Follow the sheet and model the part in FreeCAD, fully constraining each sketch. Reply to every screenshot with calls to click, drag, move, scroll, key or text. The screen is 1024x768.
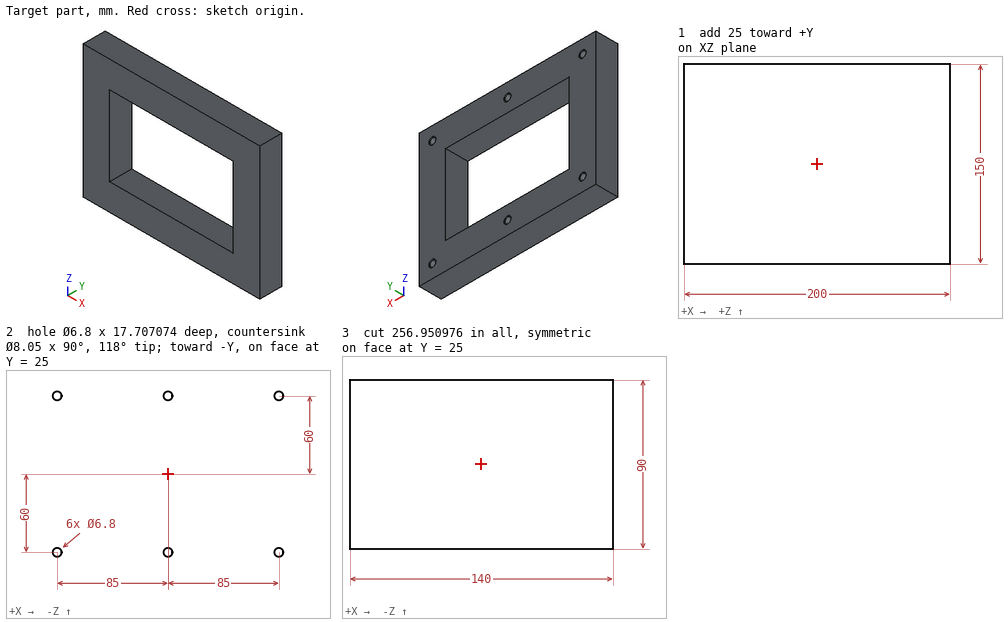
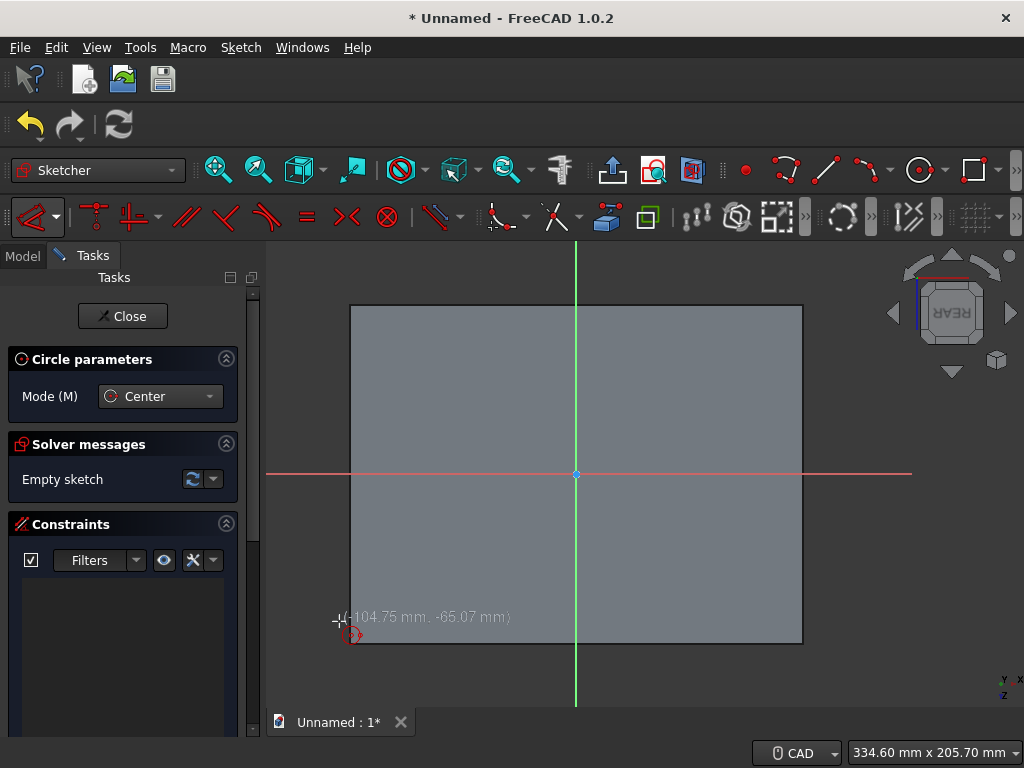
click(384, 610)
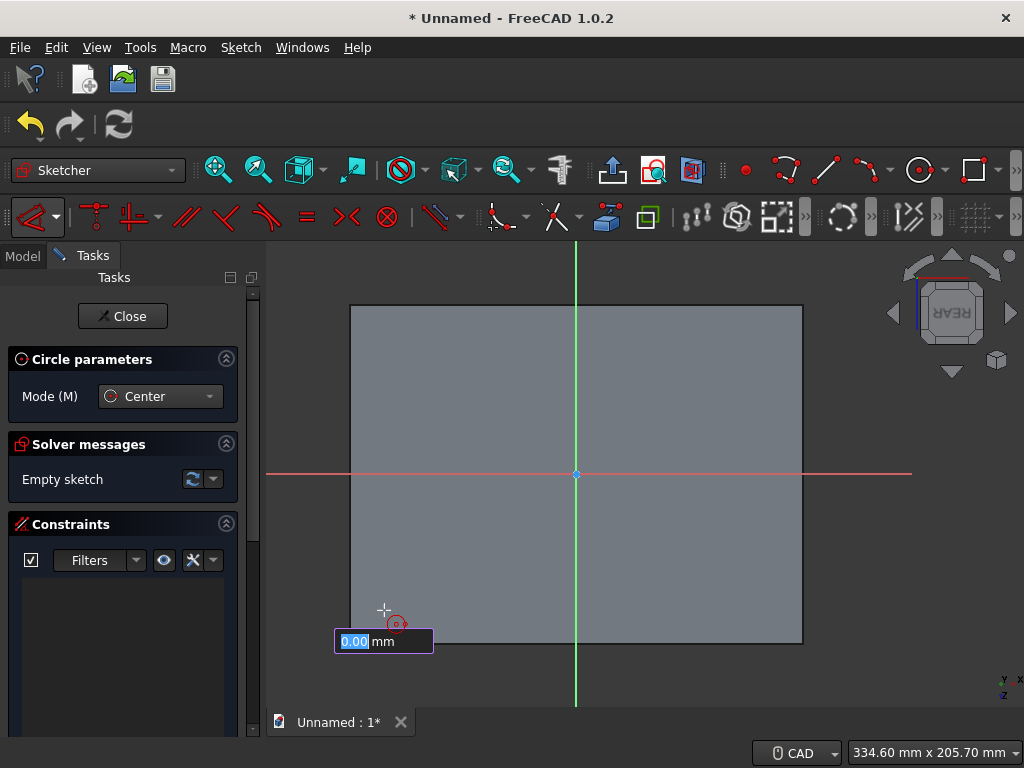
scroll(389, 605, up, 4)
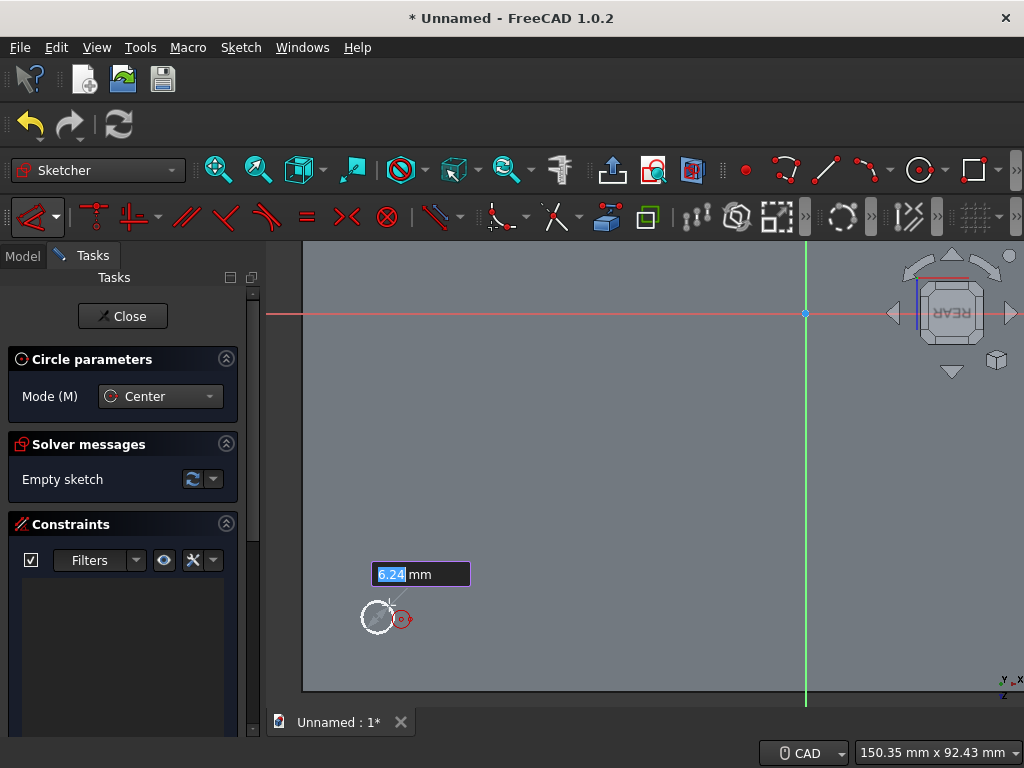
click(389, 604)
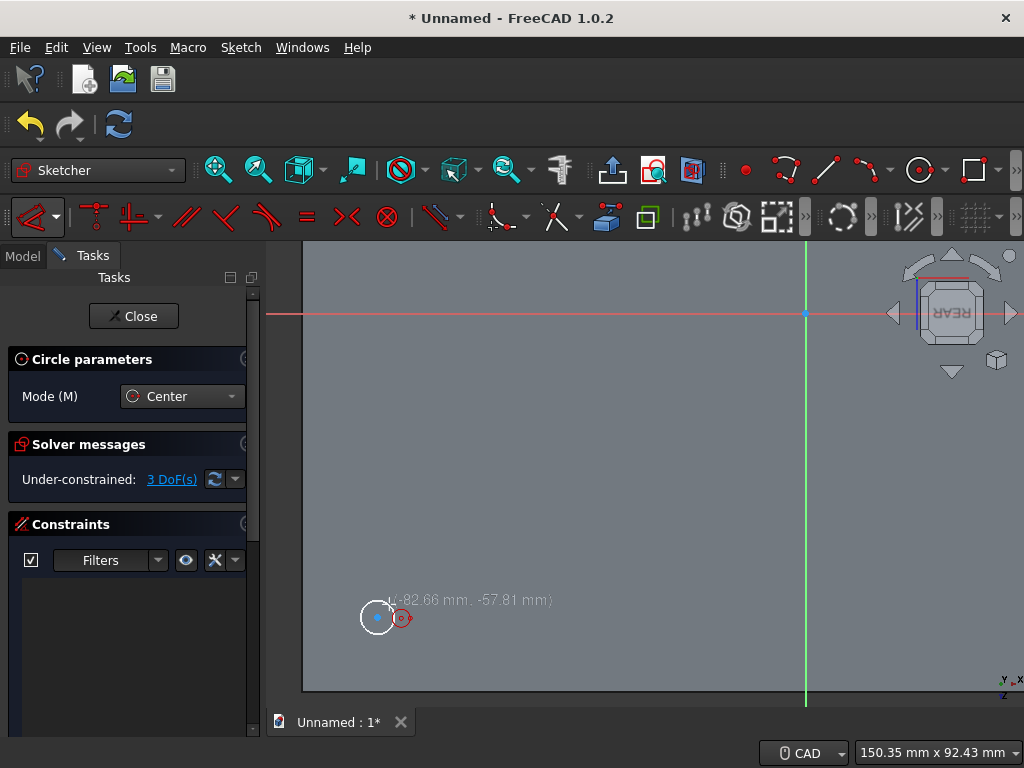
scroll(806, 616, up, 2)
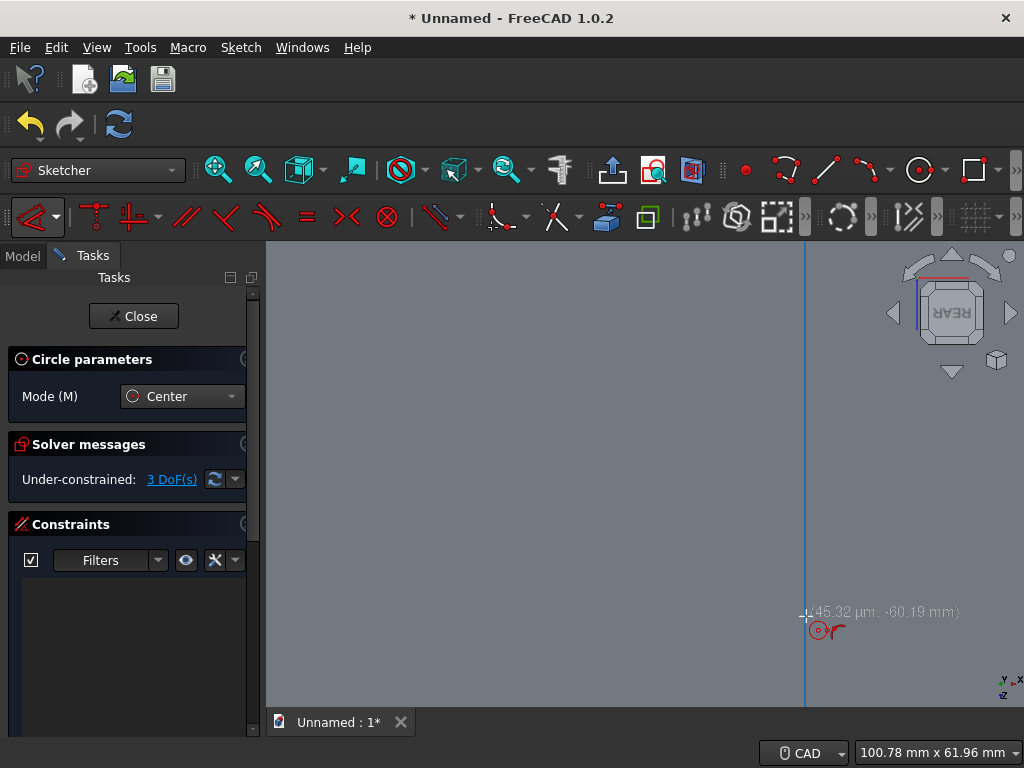
scroll(478, 607, down, 6)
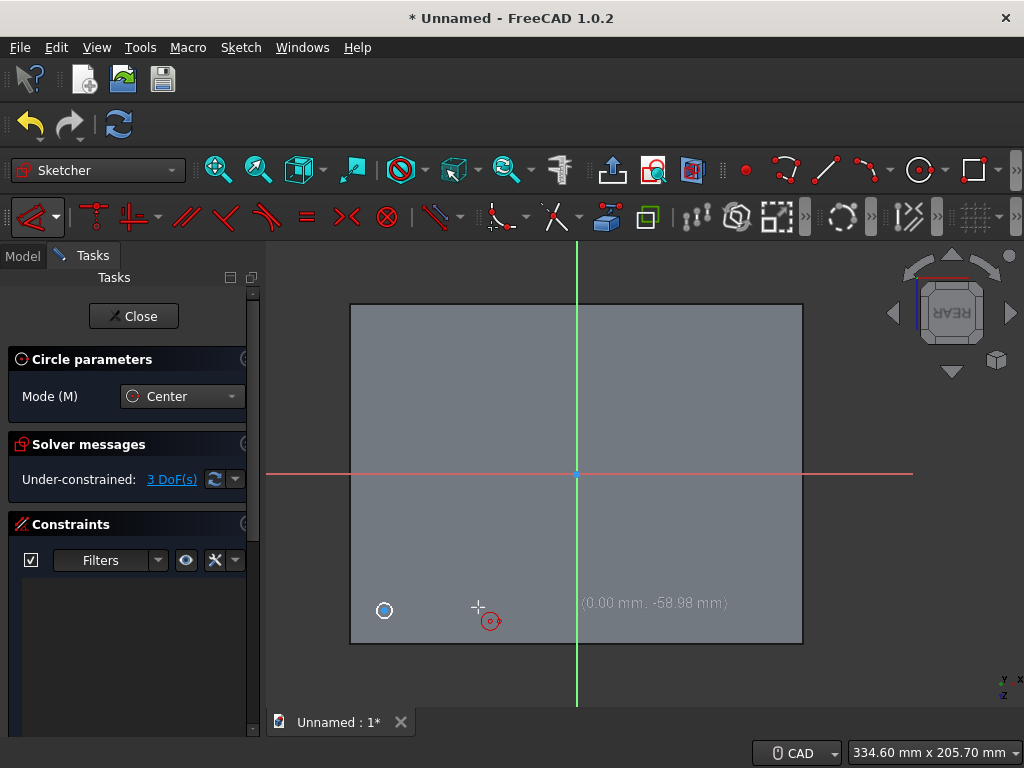
click(577, 610)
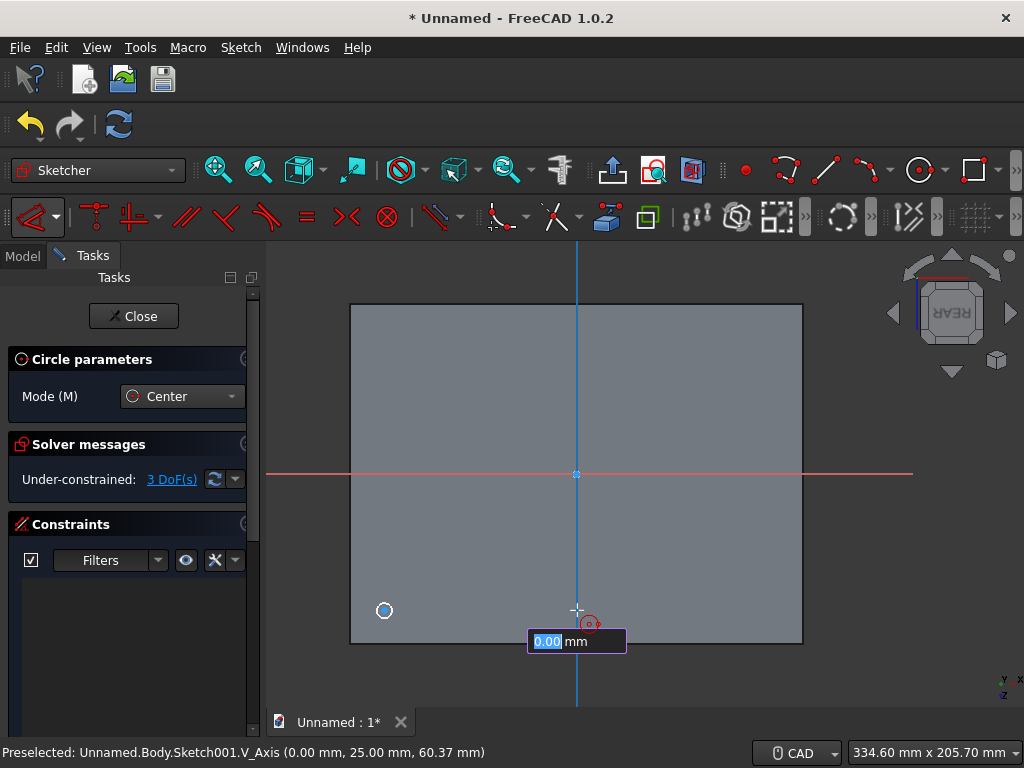
scroll(584, 608, up, 4)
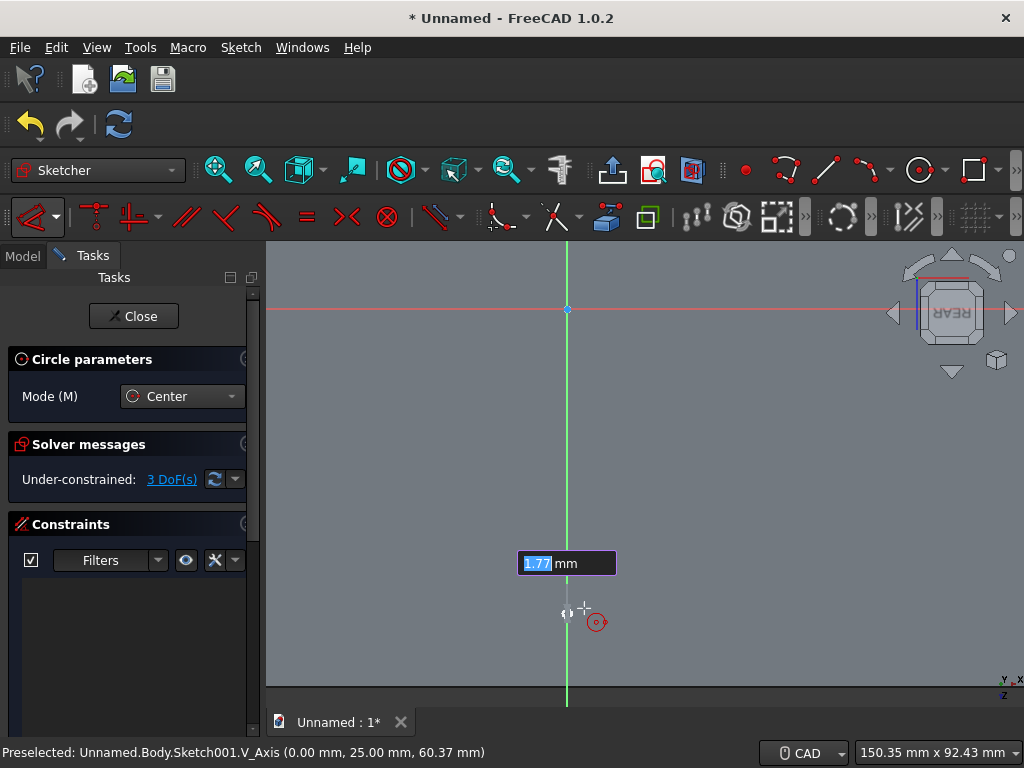
click(584, 606)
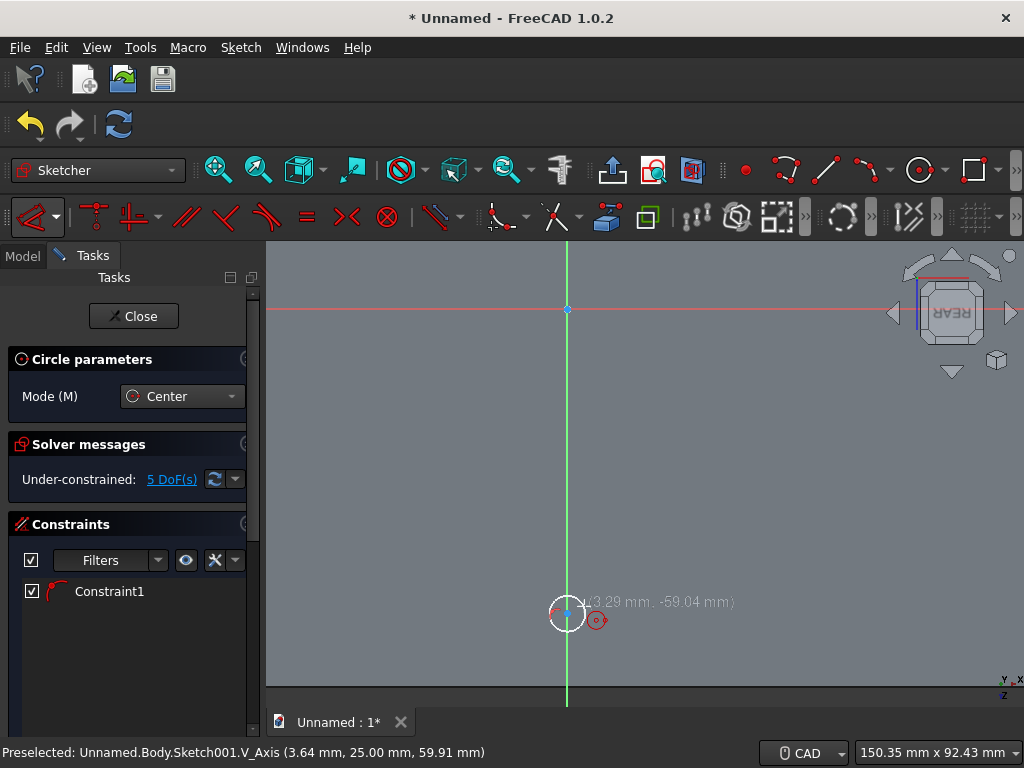
scroll(584, 608, down, 4)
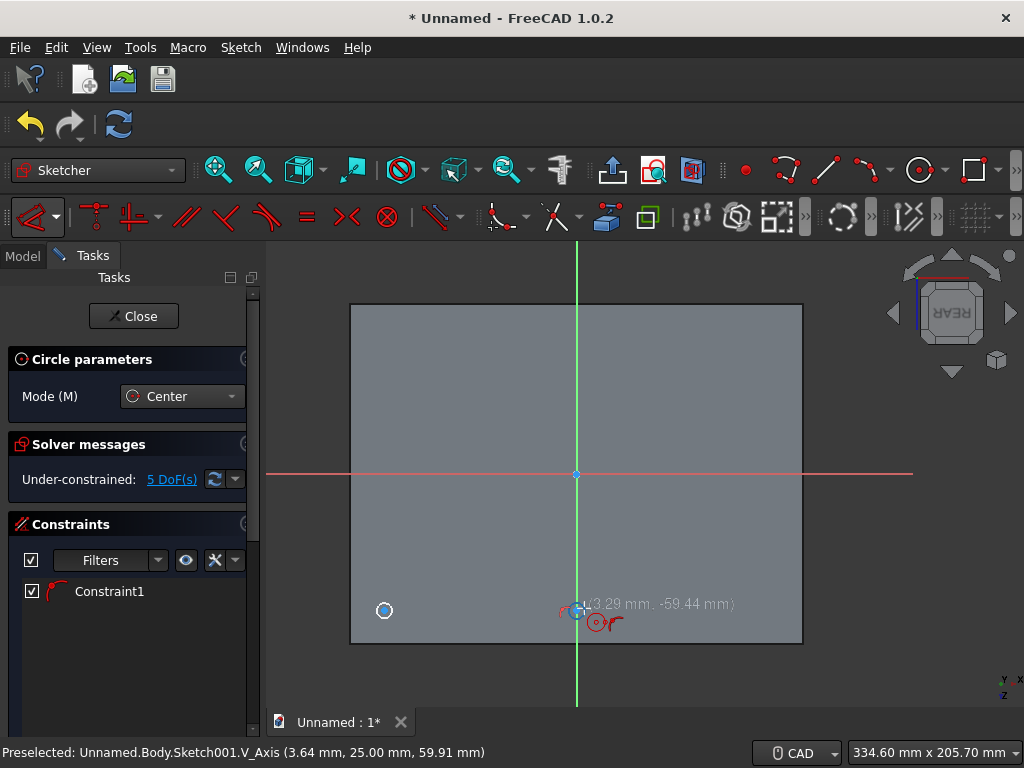
scroll(769, 610, up, 6)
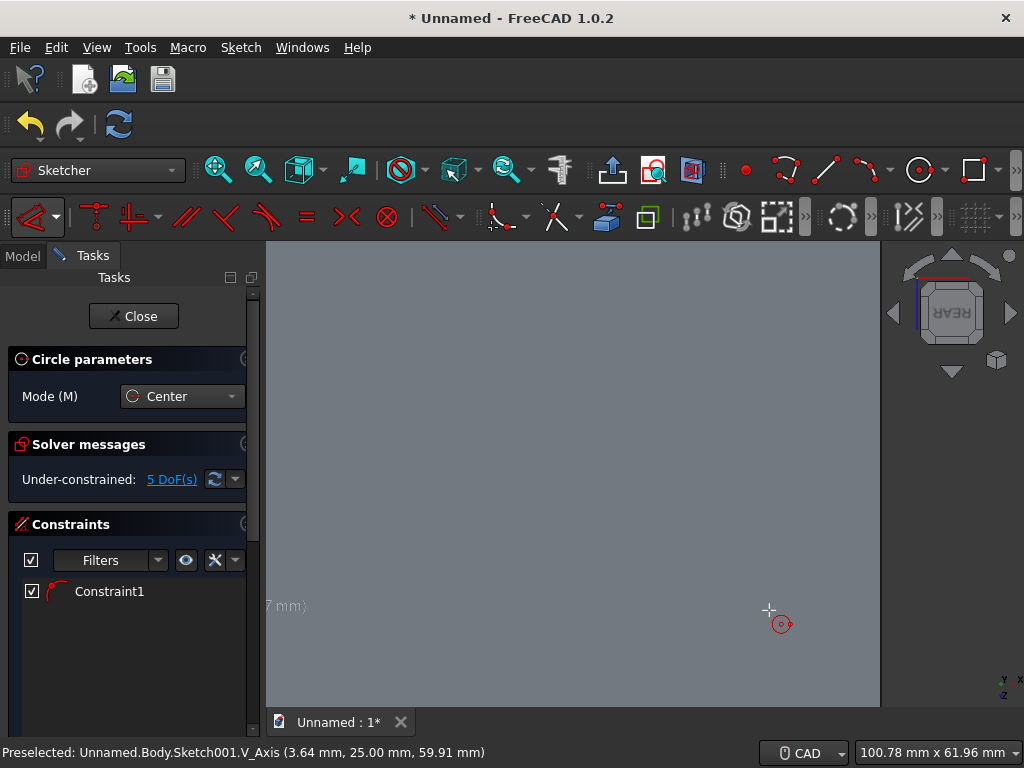
scroll(769, 610, down, 6)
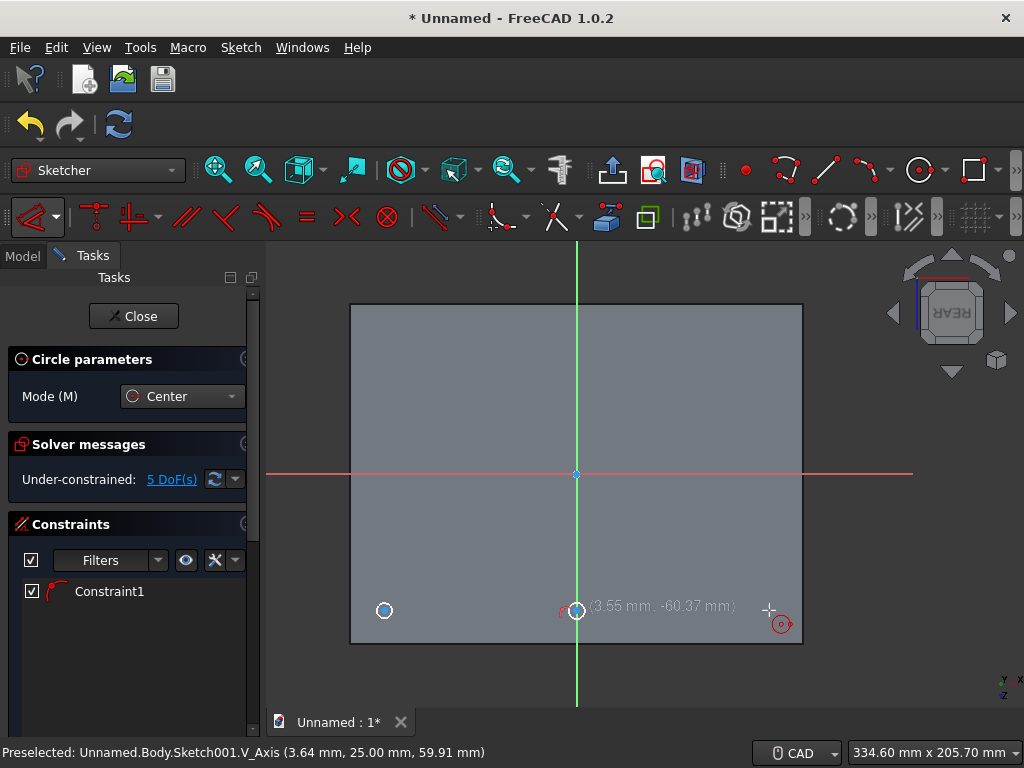
click(769, 610)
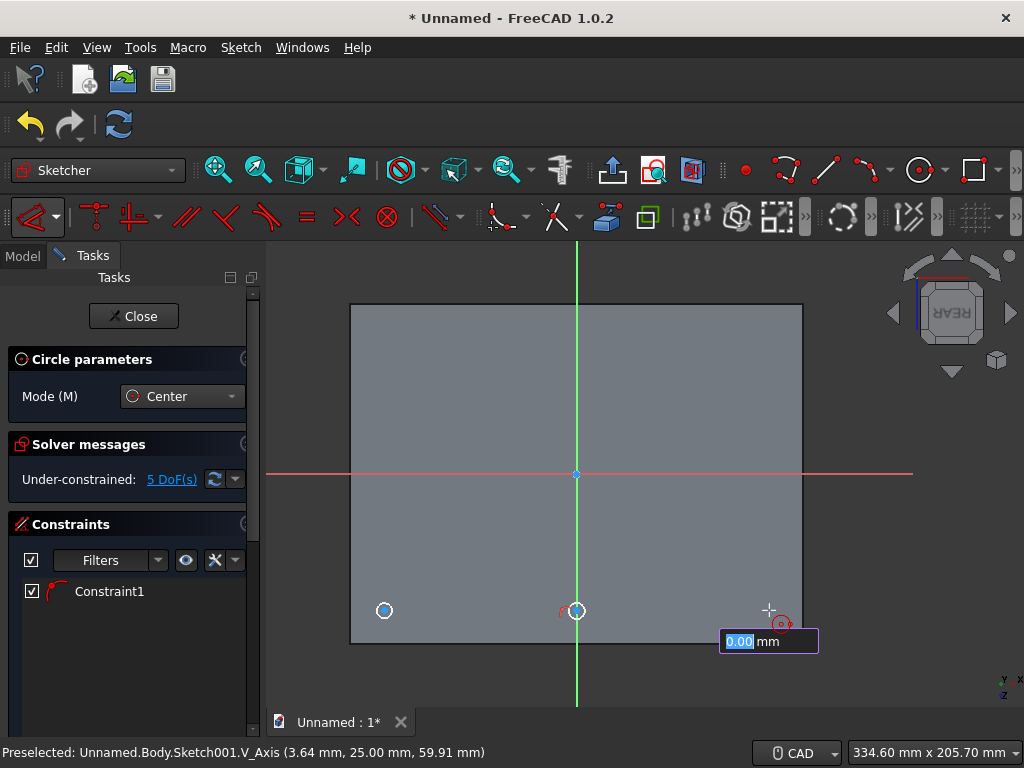
scroll(775, 605, up, 4)